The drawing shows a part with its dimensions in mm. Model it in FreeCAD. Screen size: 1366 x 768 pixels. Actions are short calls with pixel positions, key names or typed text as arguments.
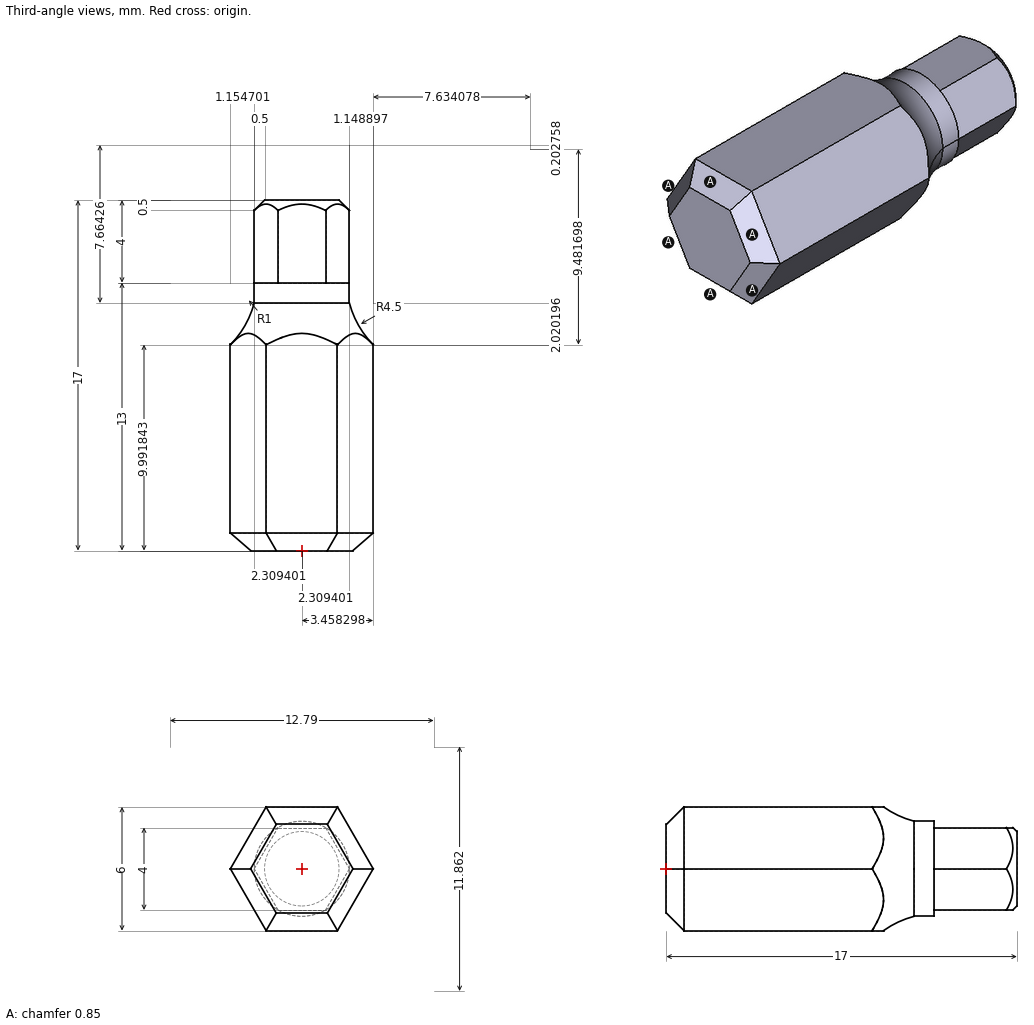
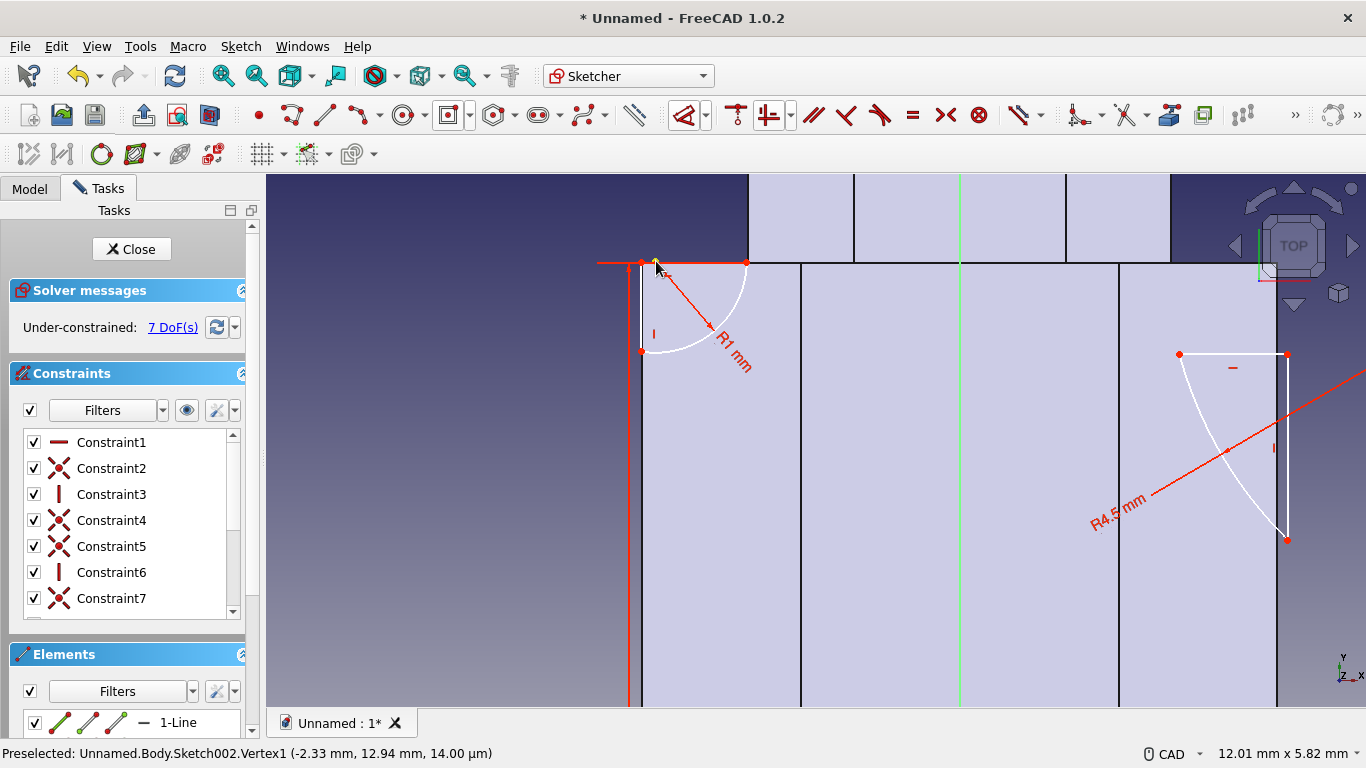
click(655, 261)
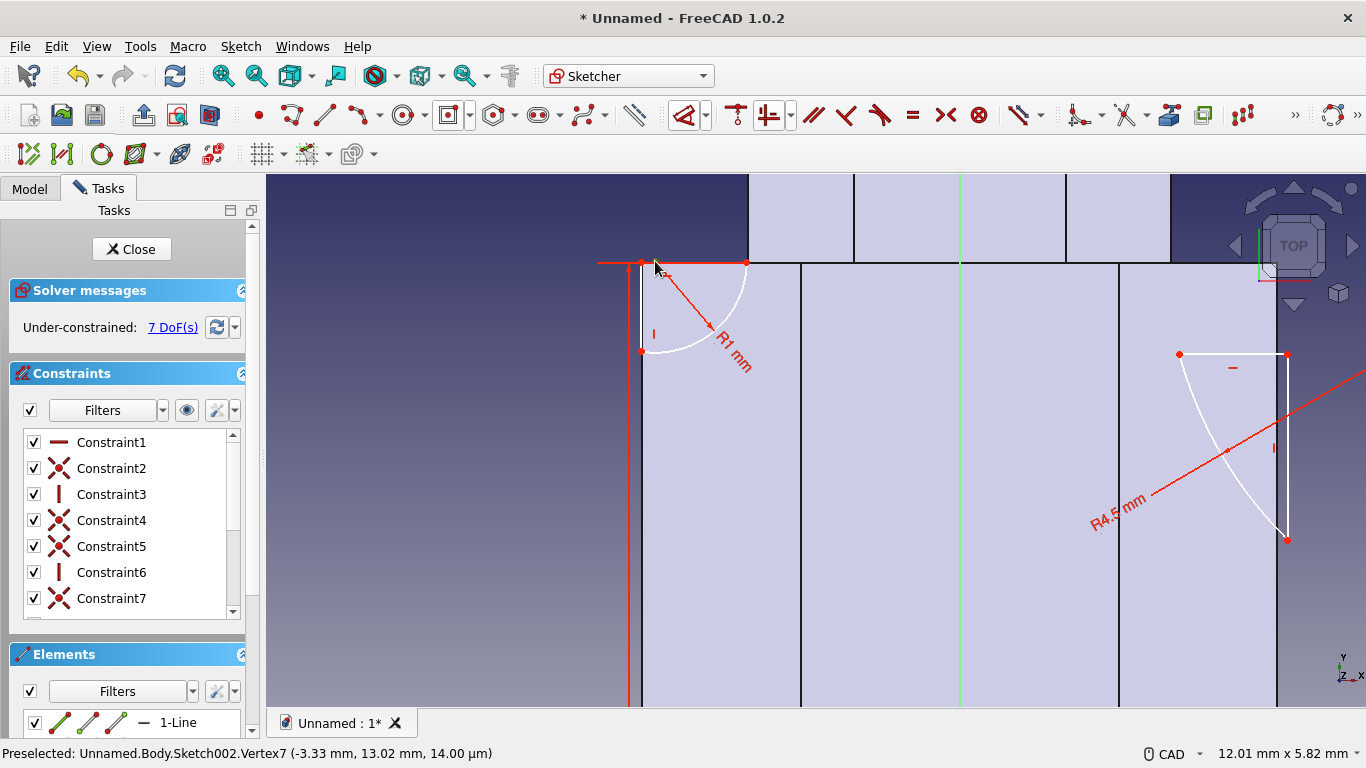
click(706, 116)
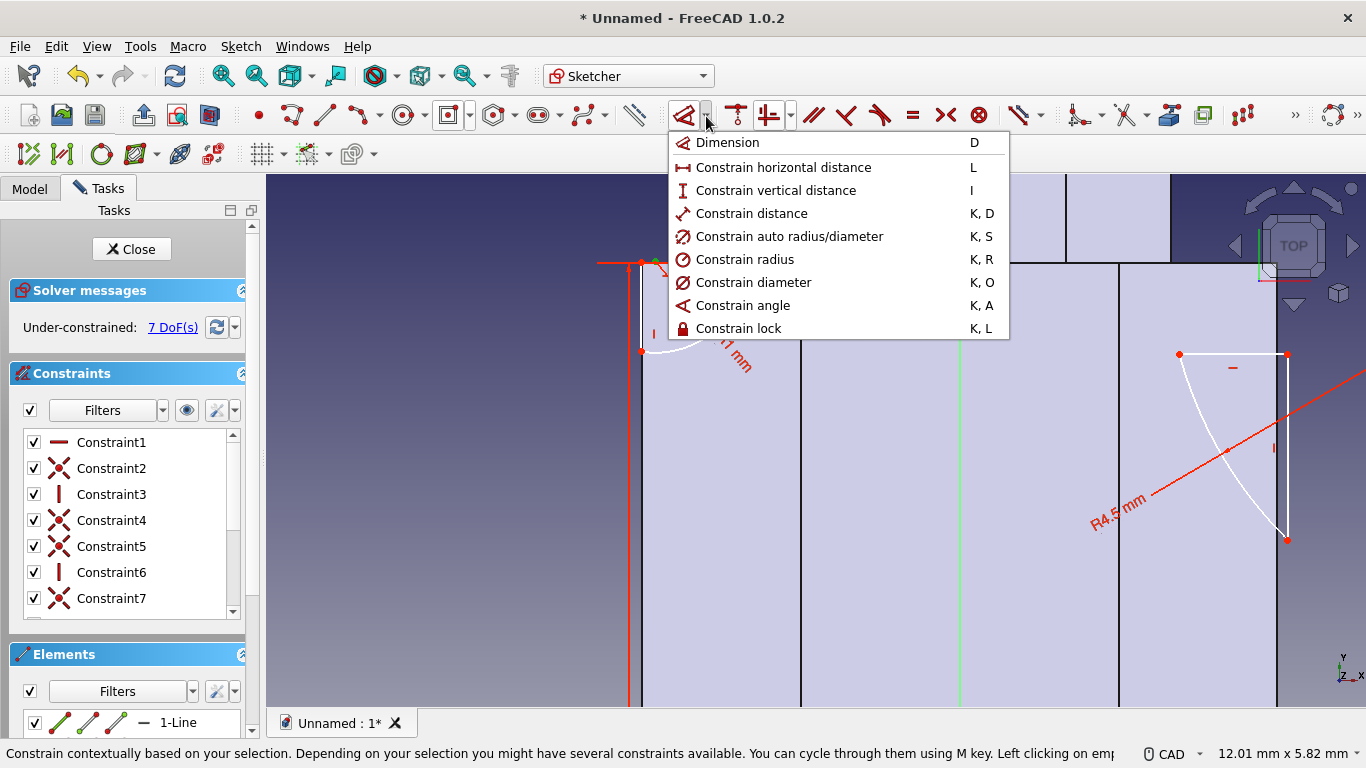
click(839, 190)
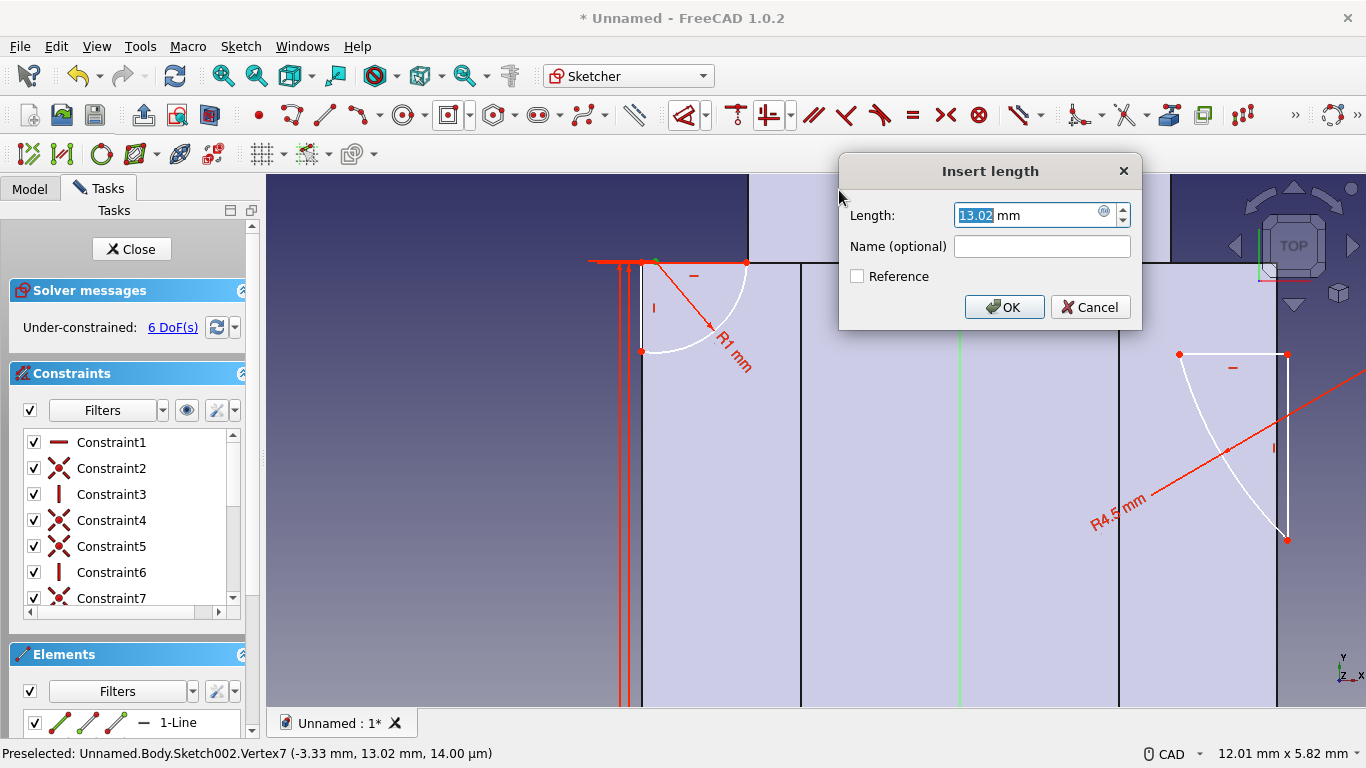
text(13)
key(Return)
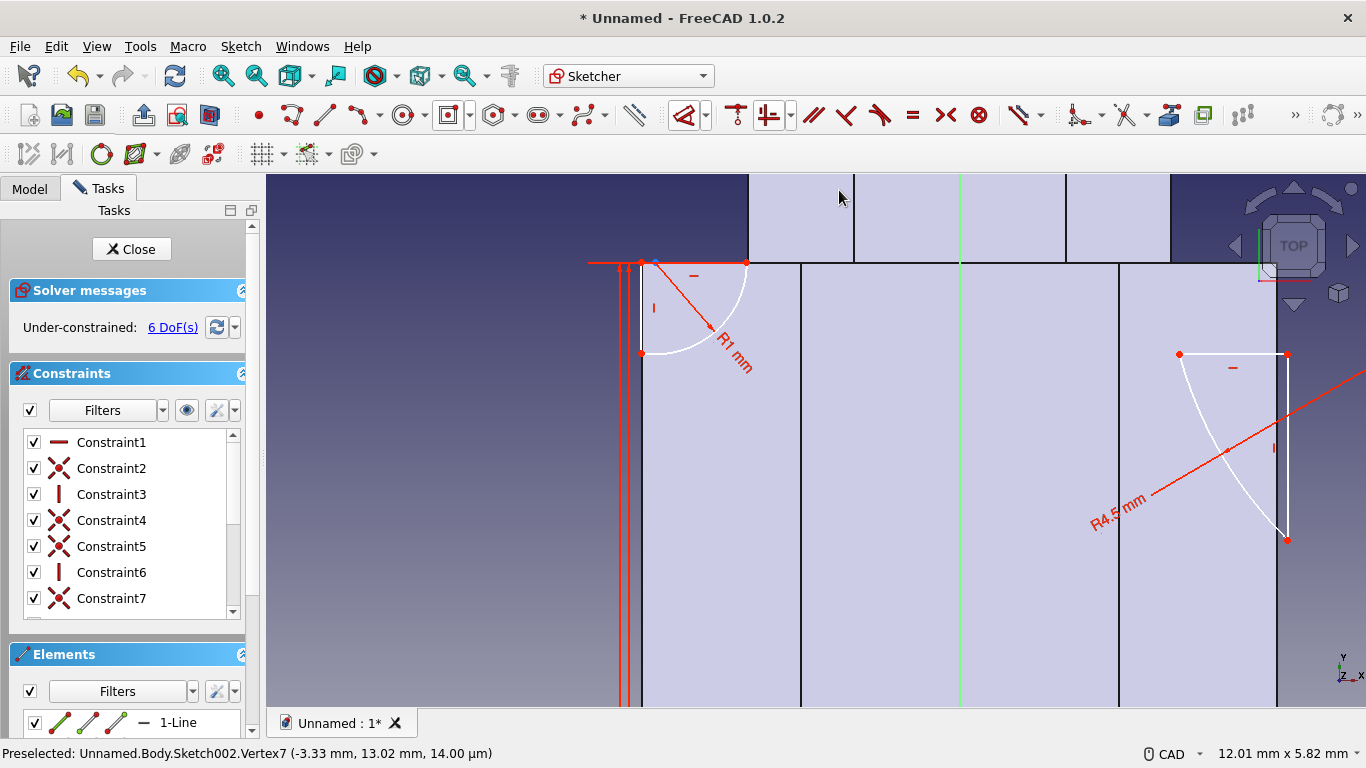
click(715, 263)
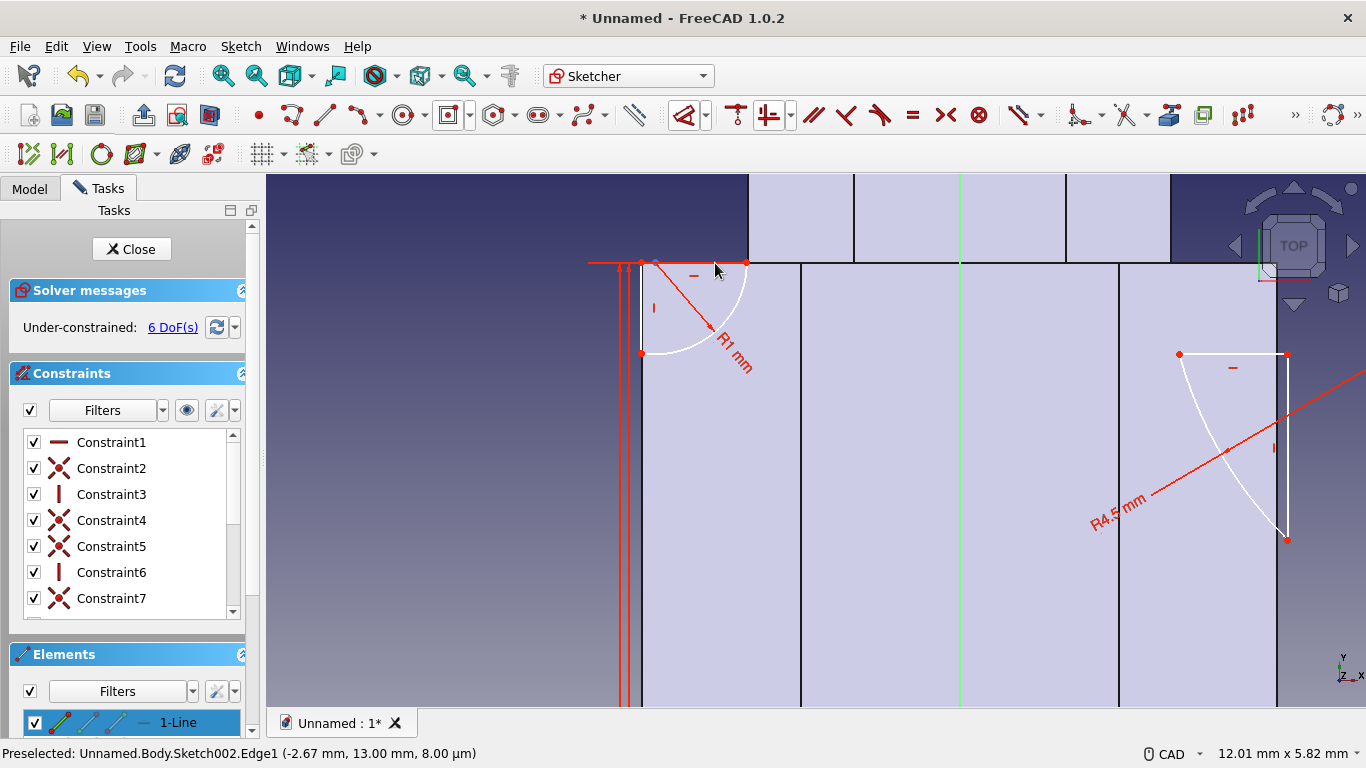
key(l)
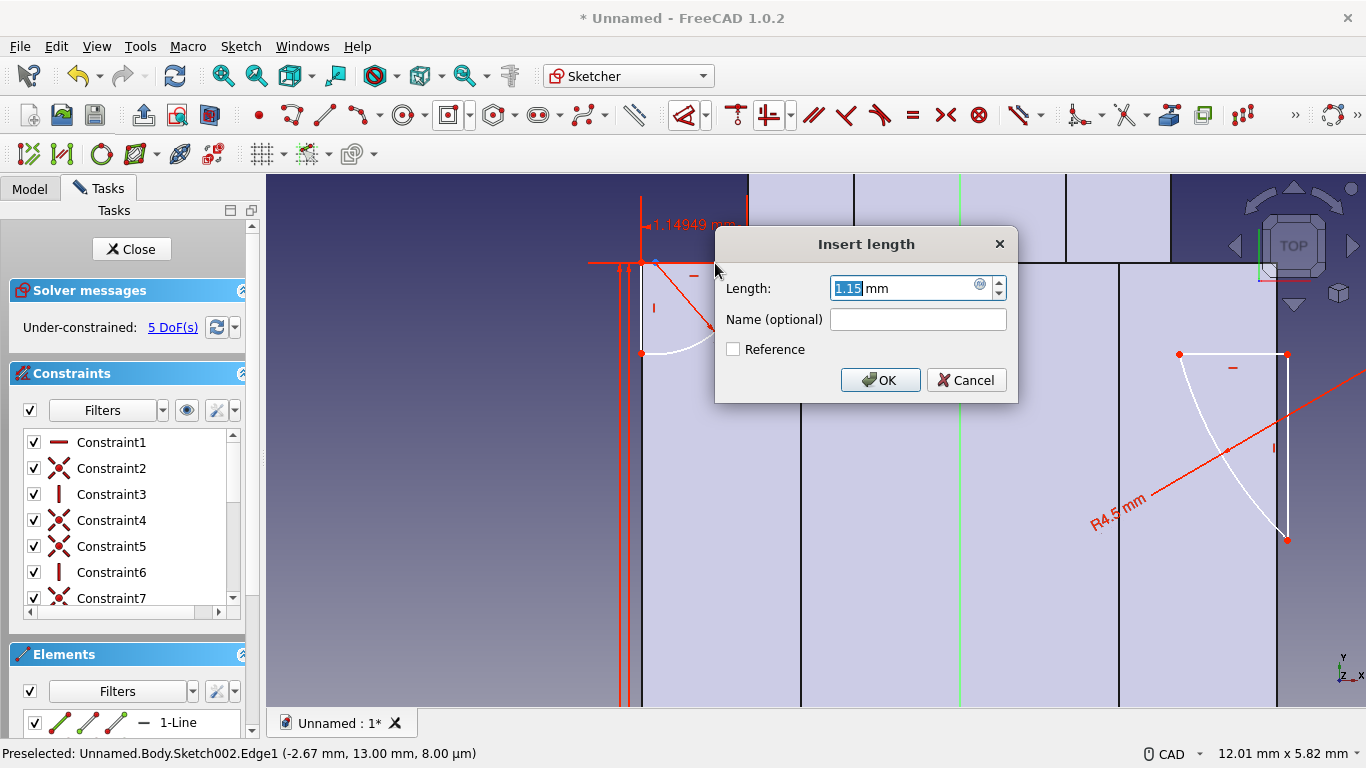
text(1.154701)
key(Return)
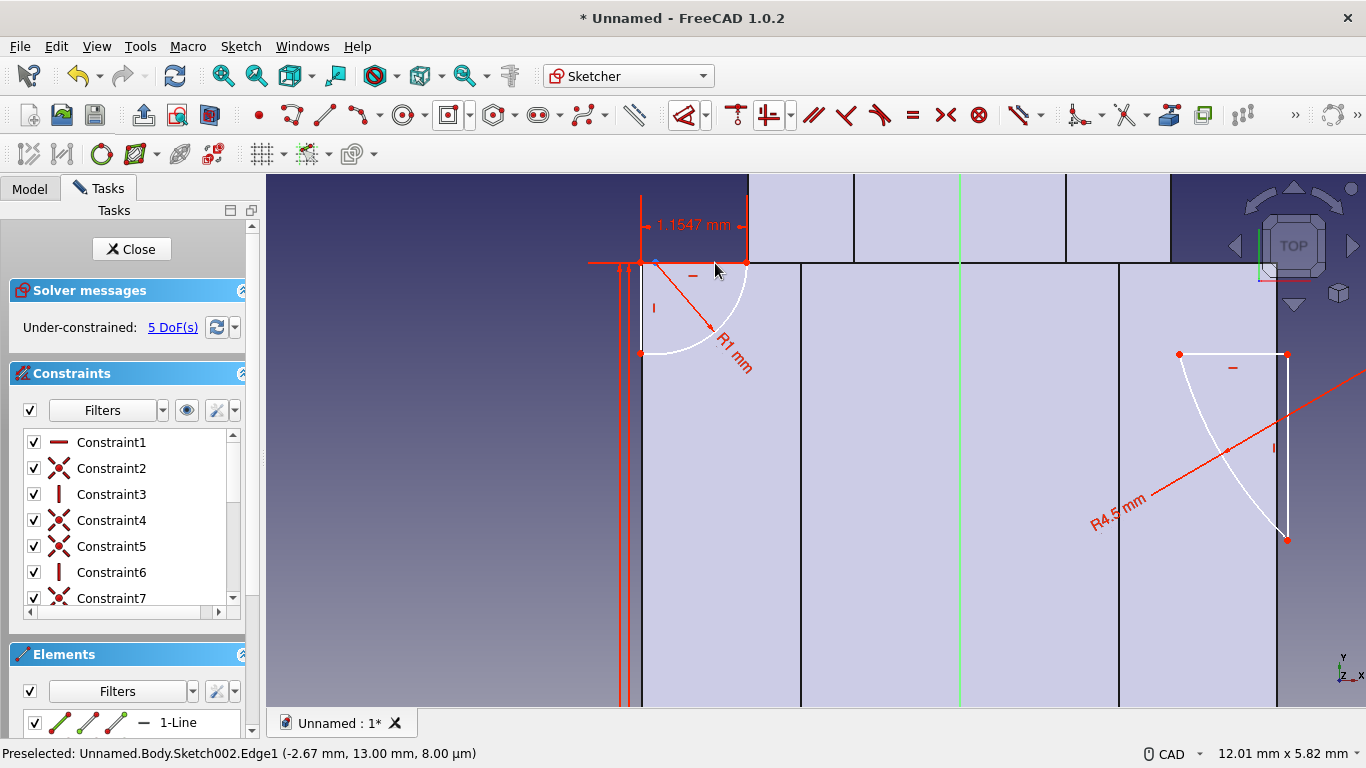
scroll(656, 260, down, 6)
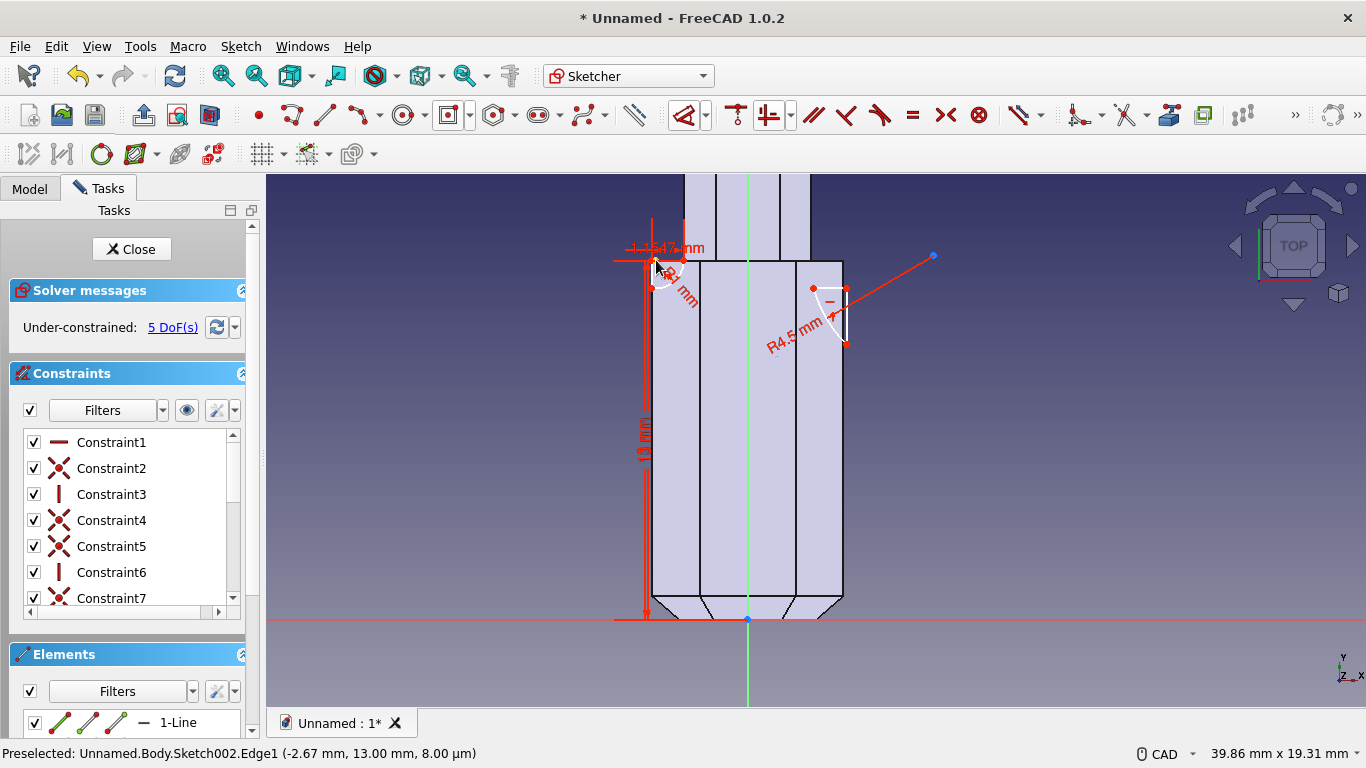
click(847, 328)